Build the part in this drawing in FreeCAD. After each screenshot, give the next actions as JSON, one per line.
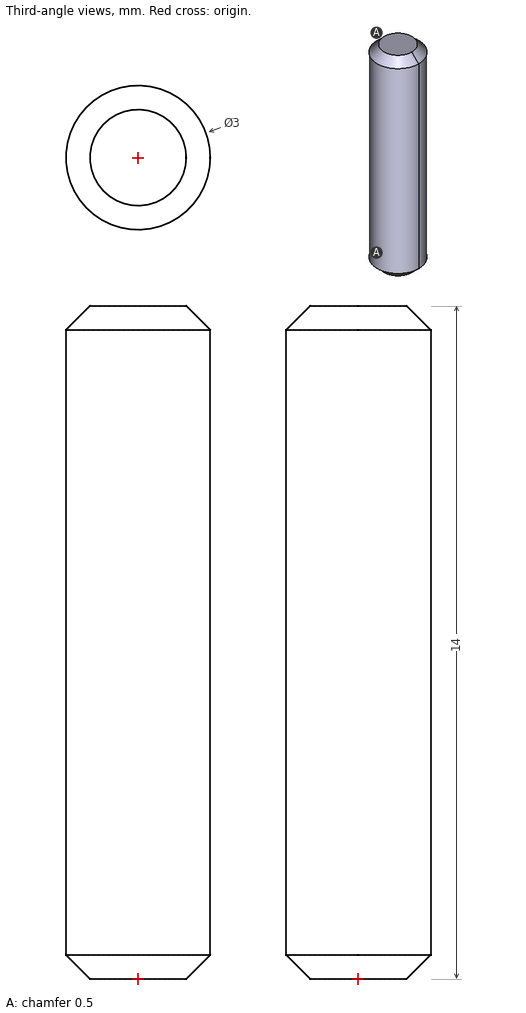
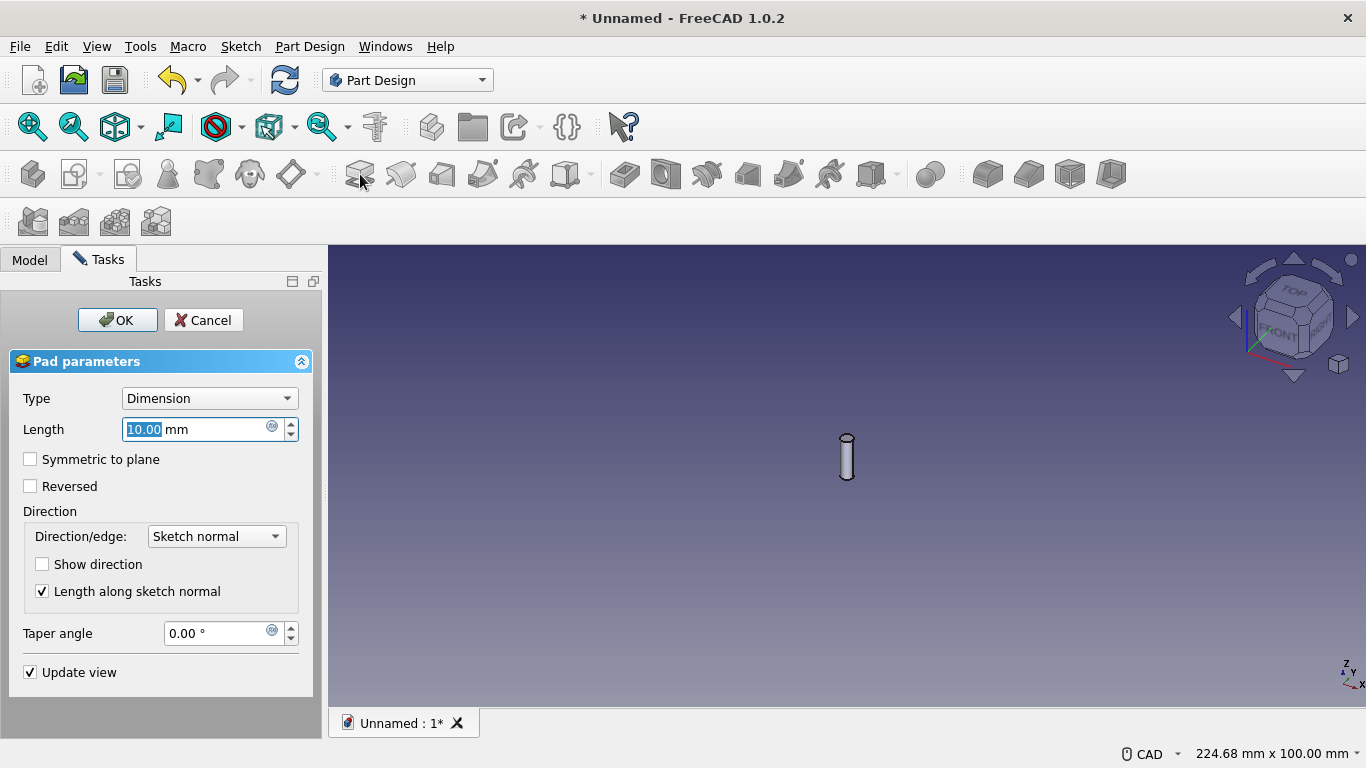
{"action": "type", "text": "14"}
{"action": "key", "text": "Tab"}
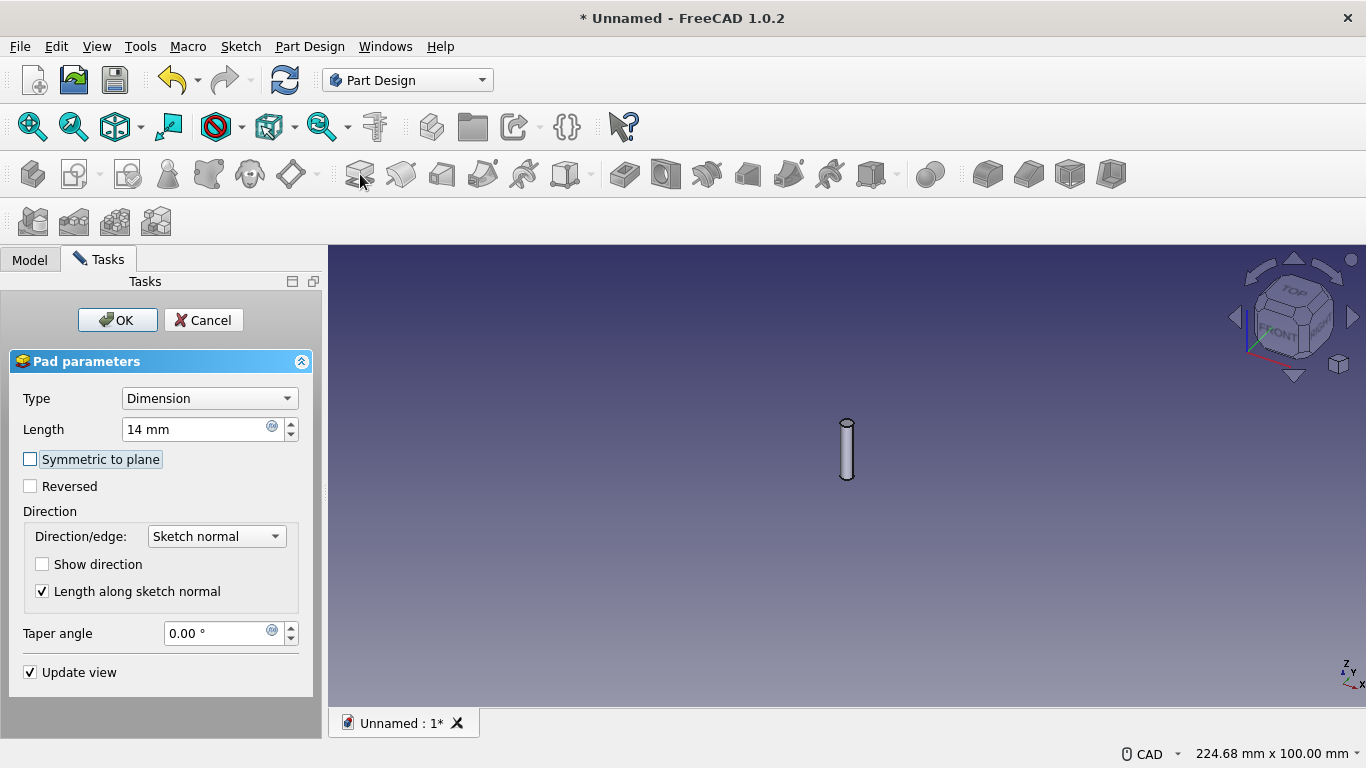
{"action": "left_click", "coordinate": [118, 320]}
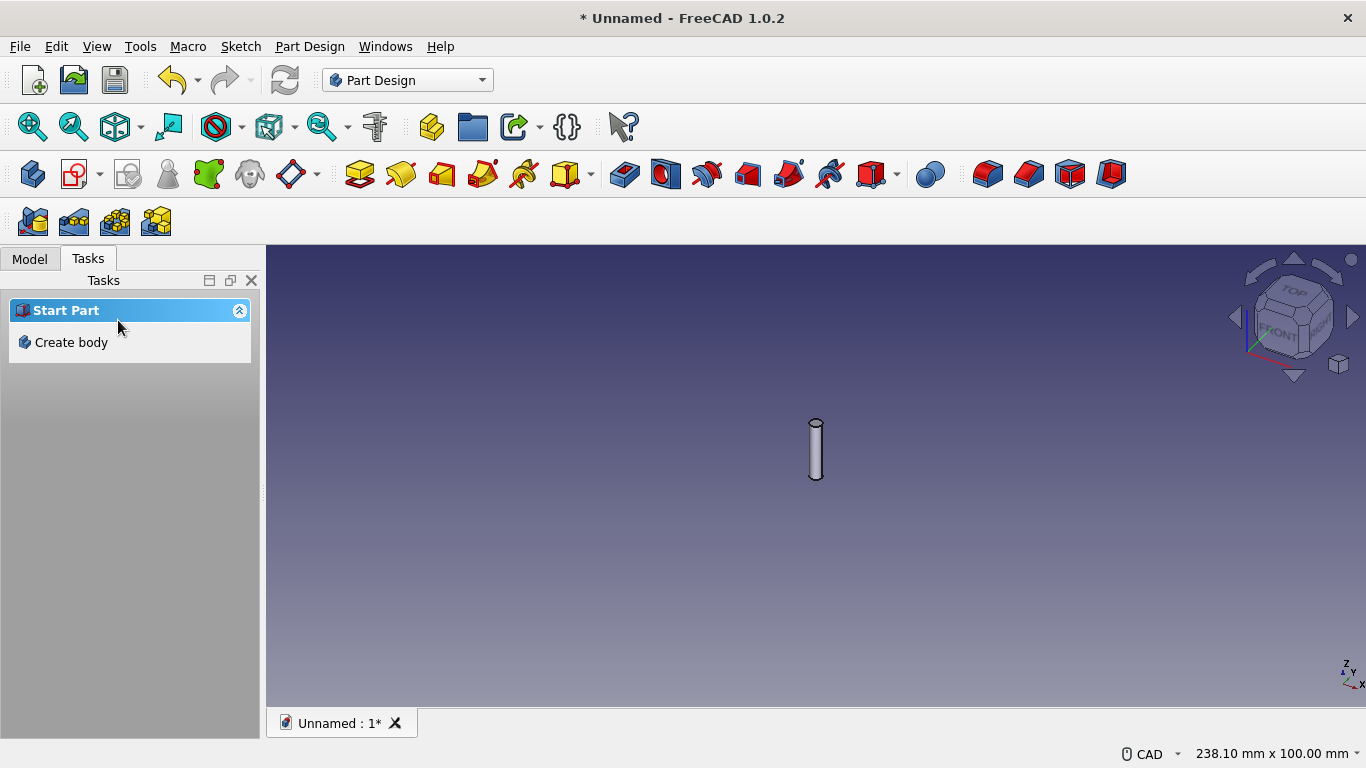
{"action": "left_click", "coordinate": [33, 128]}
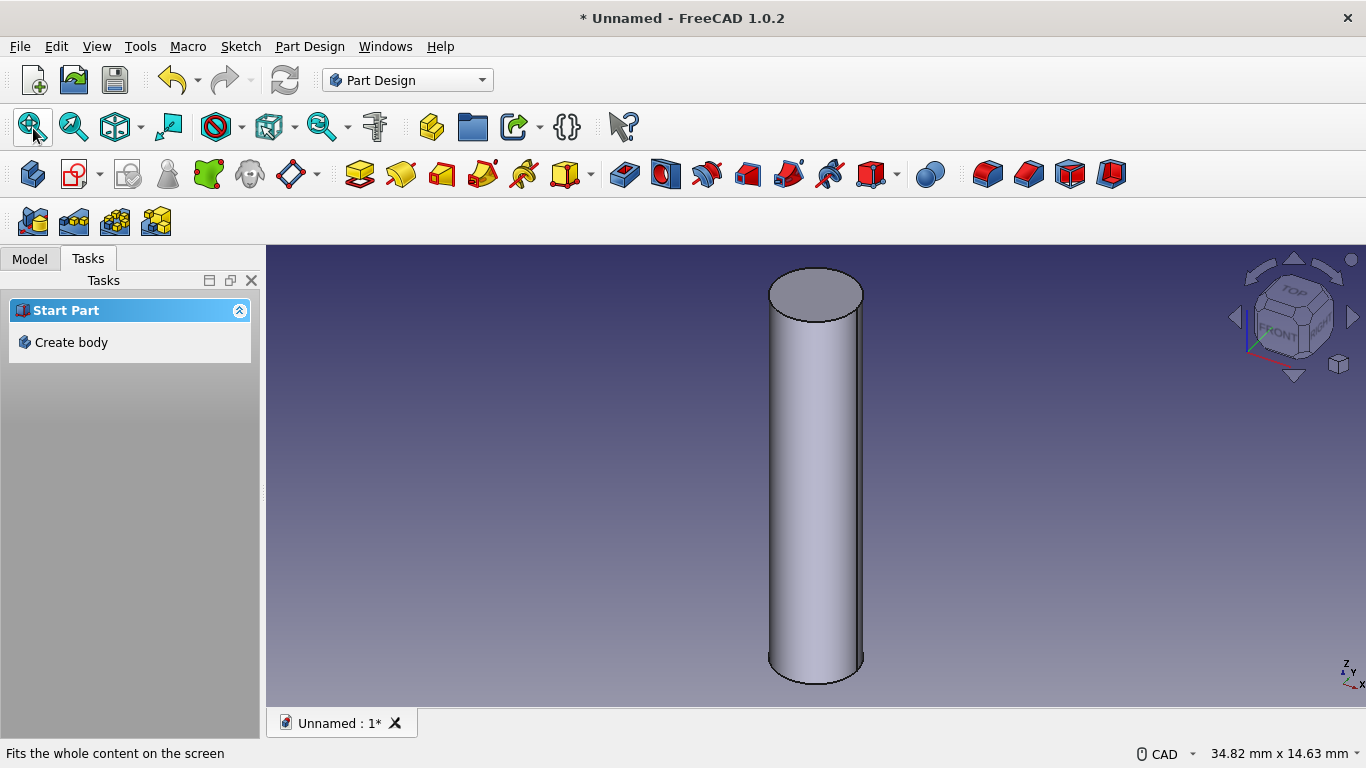
{"action": "left_click", "coordinate": [769, 297]}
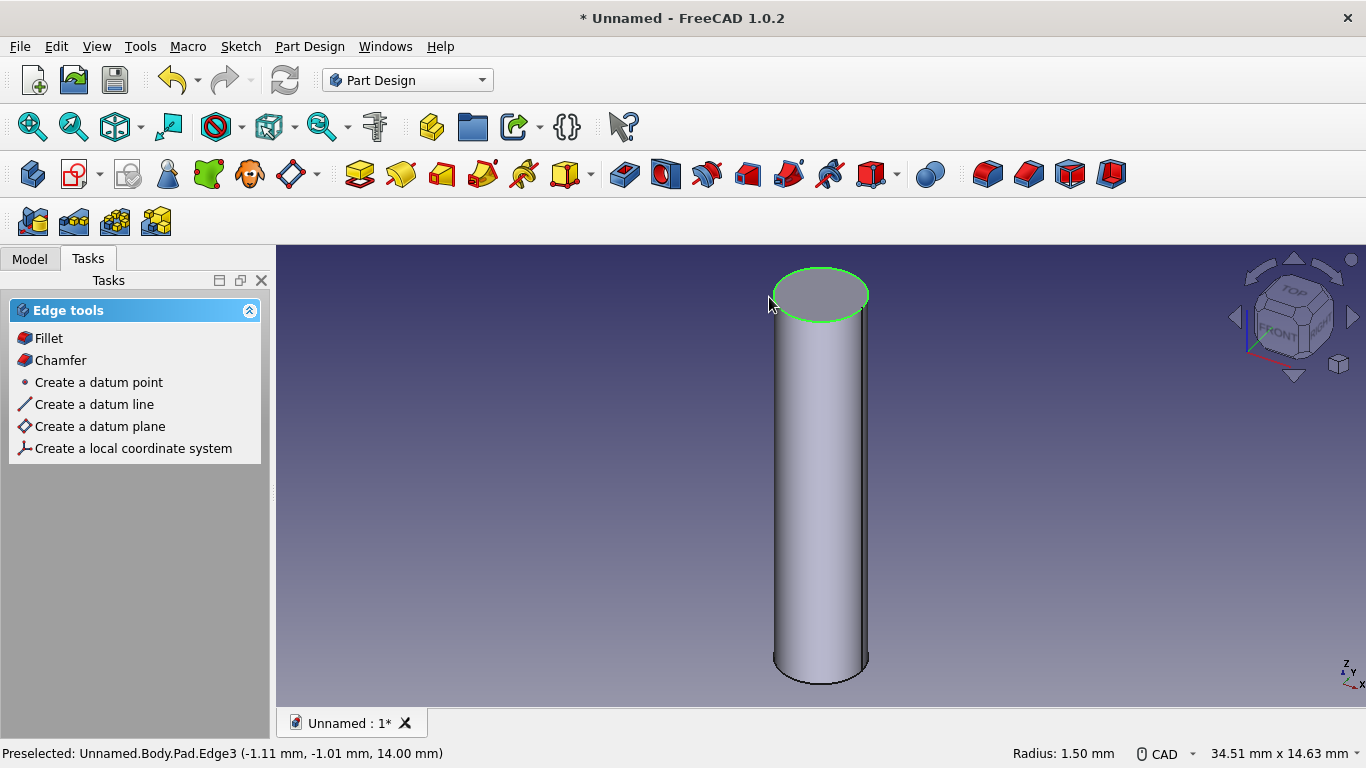
{"action": "key", "text": "0"}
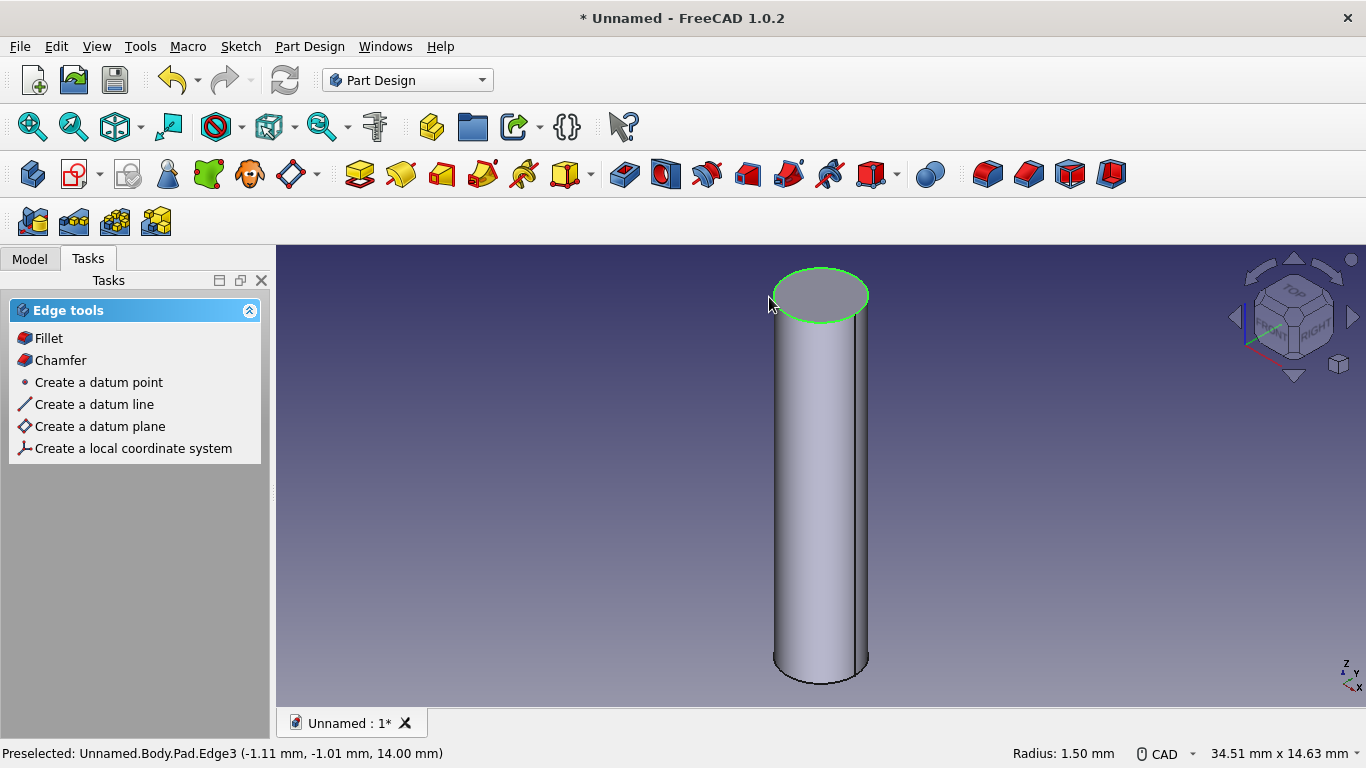
{"action": "key", "text": "2"}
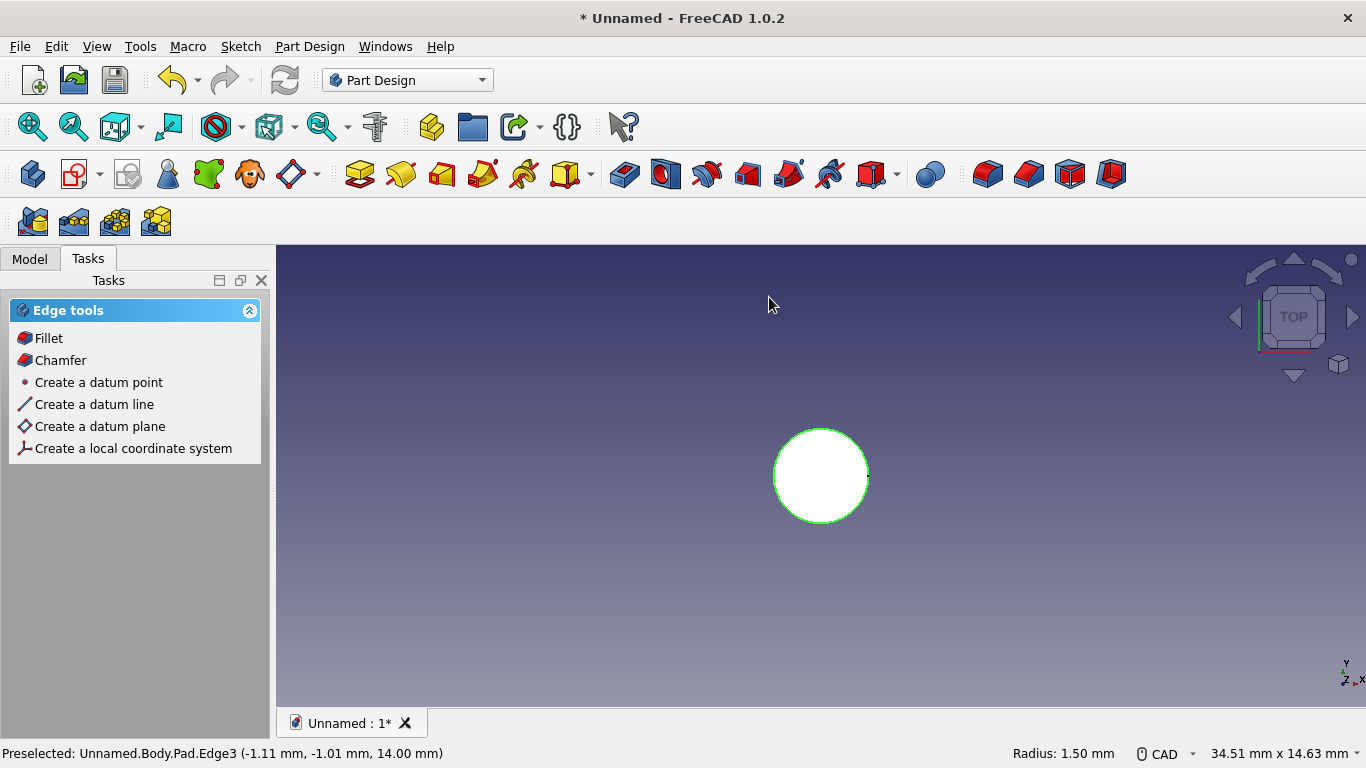
{"action": "left_click", "coordinate": [33, 128]}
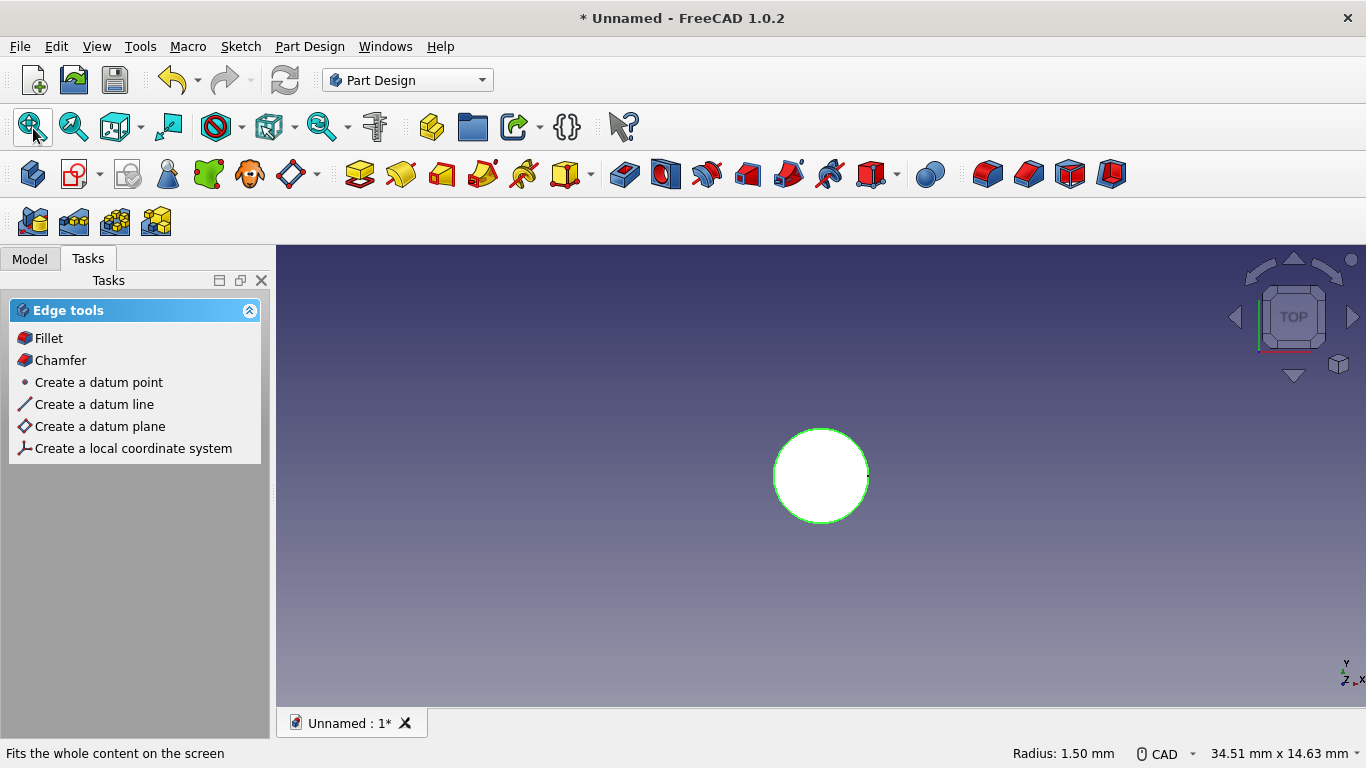
{"action": "key", "text": "1"}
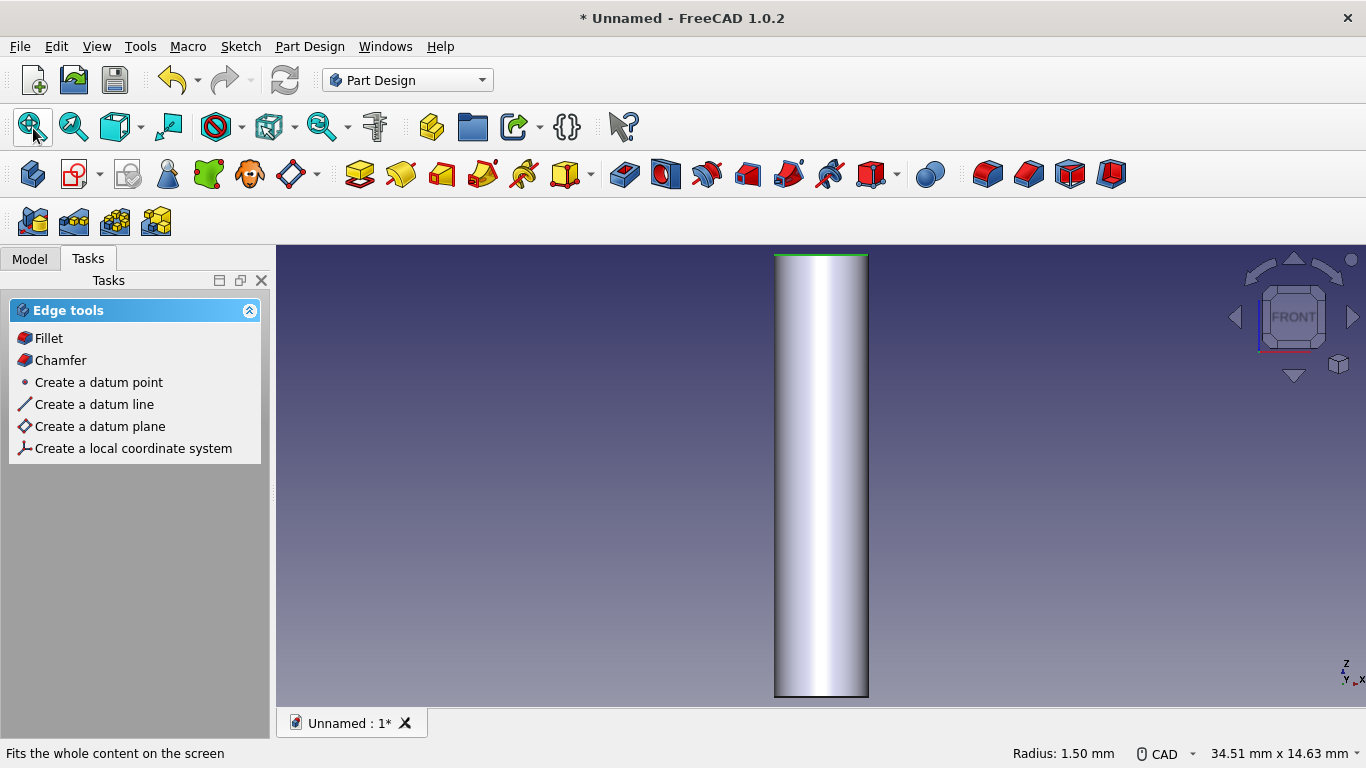
{"action": "key", "text": "3"}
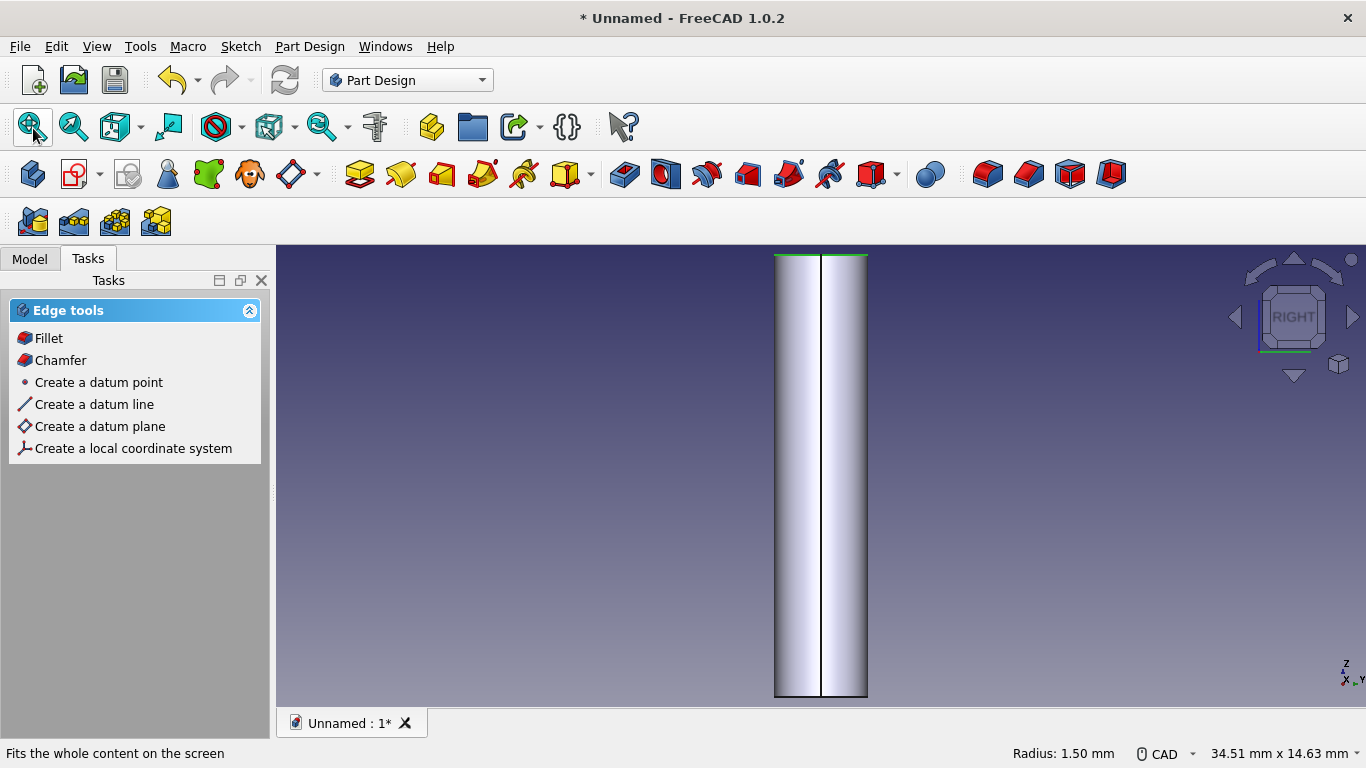
{"action": "key", "text": "5"}